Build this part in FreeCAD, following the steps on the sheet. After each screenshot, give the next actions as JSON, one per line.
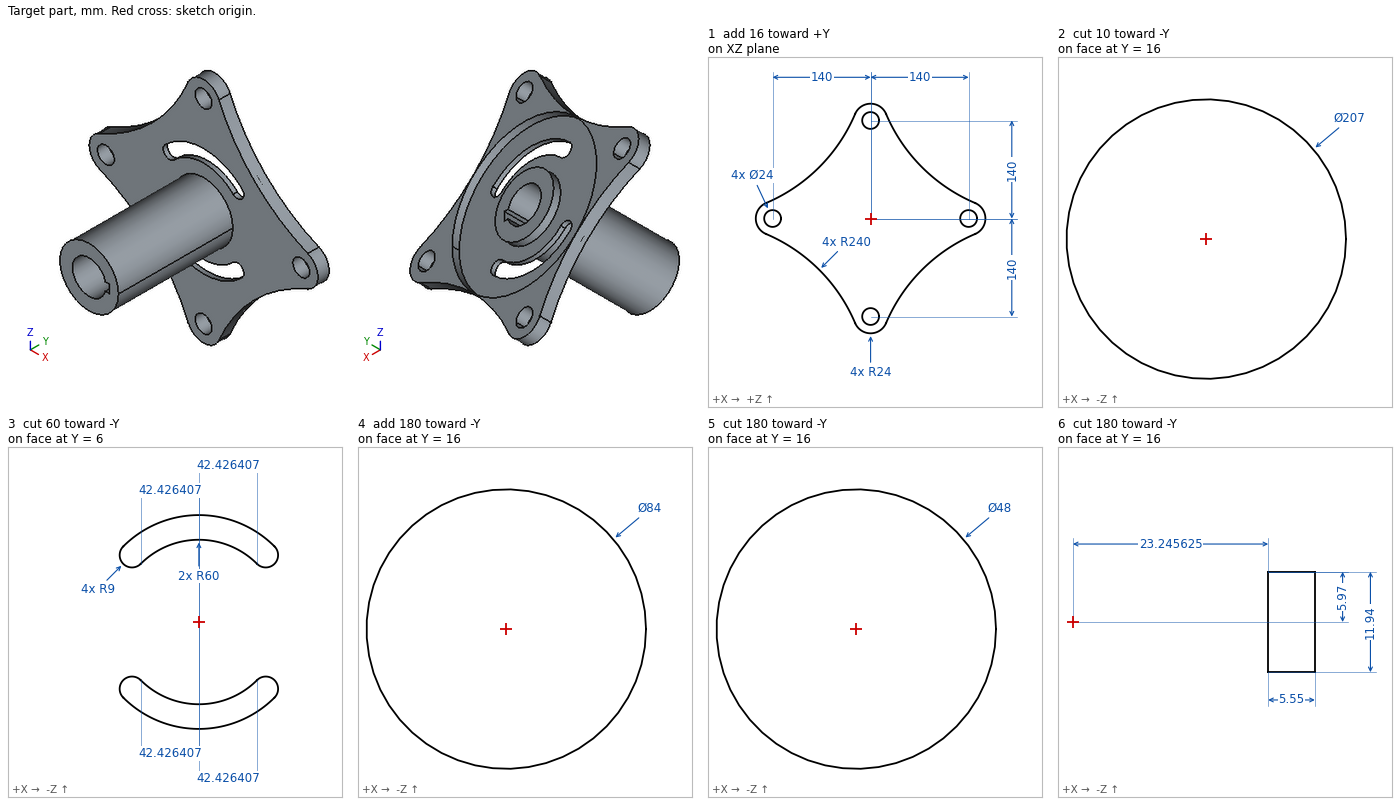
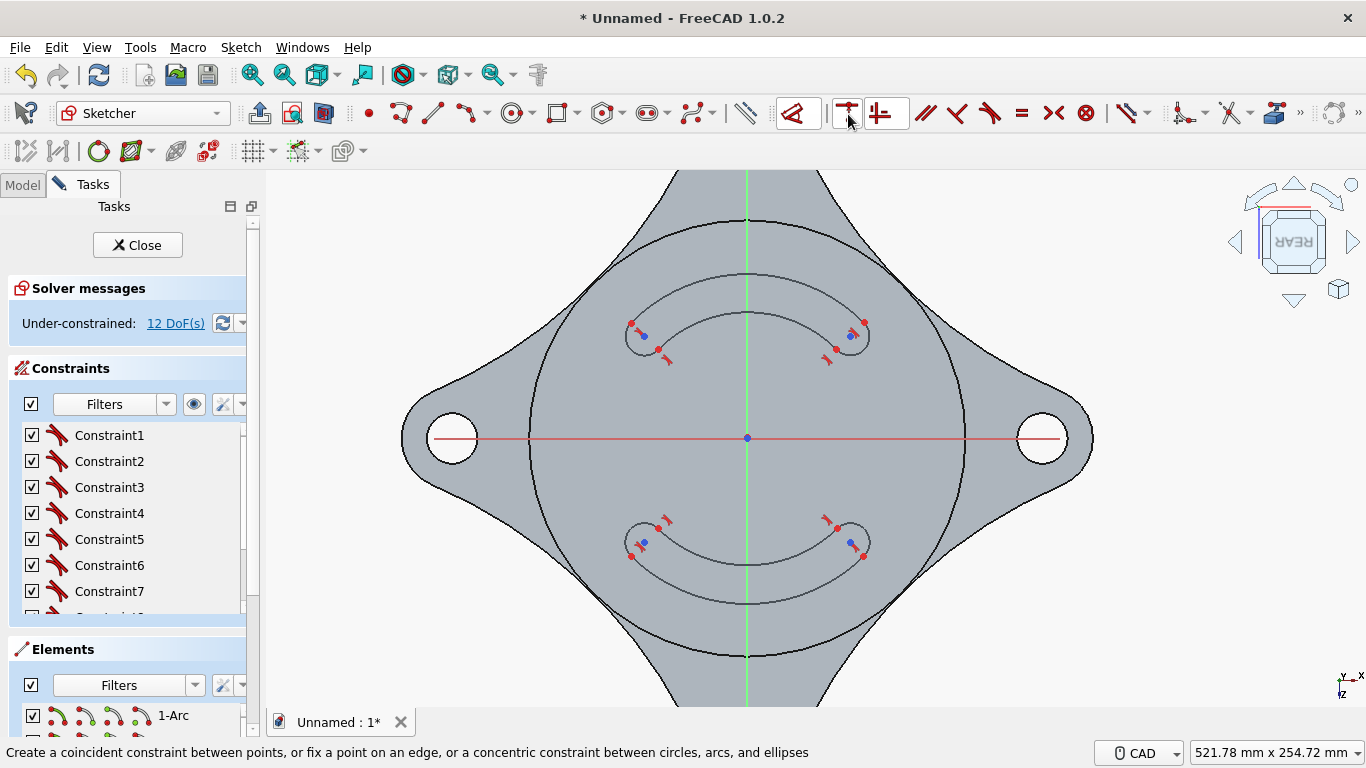
{"action": "left_click", "coordinate": [787, 319]}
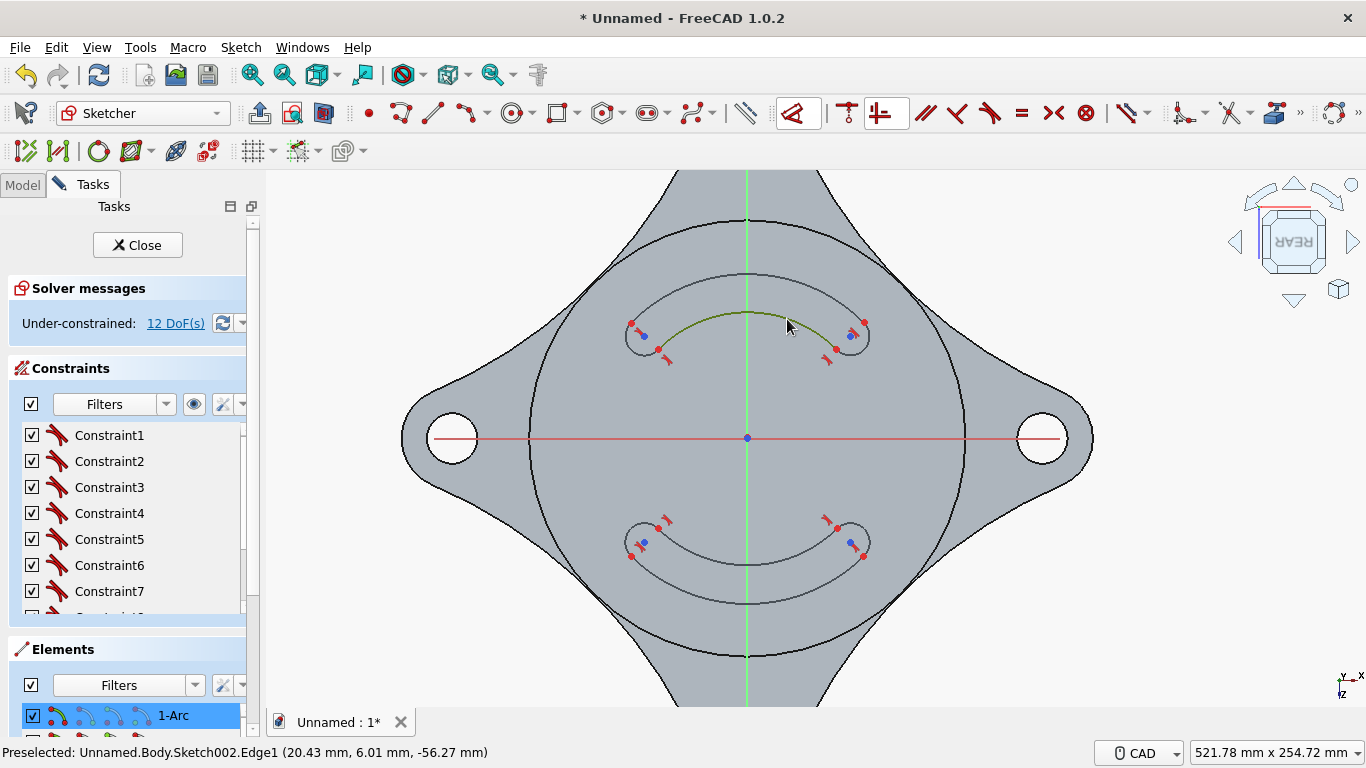
{"action": "left_click", "coordinate": [697, 596]}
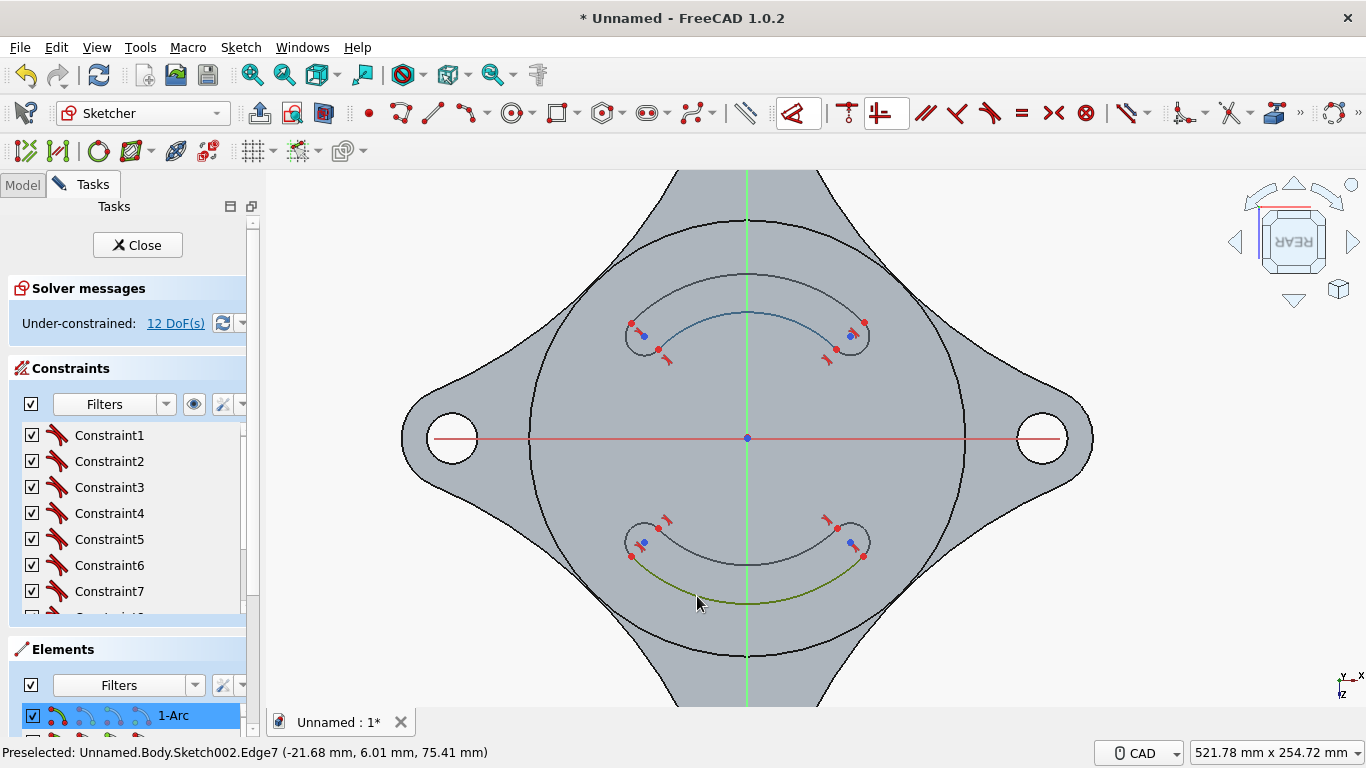
{"action": "left_click", "coordinate": [848, 114]}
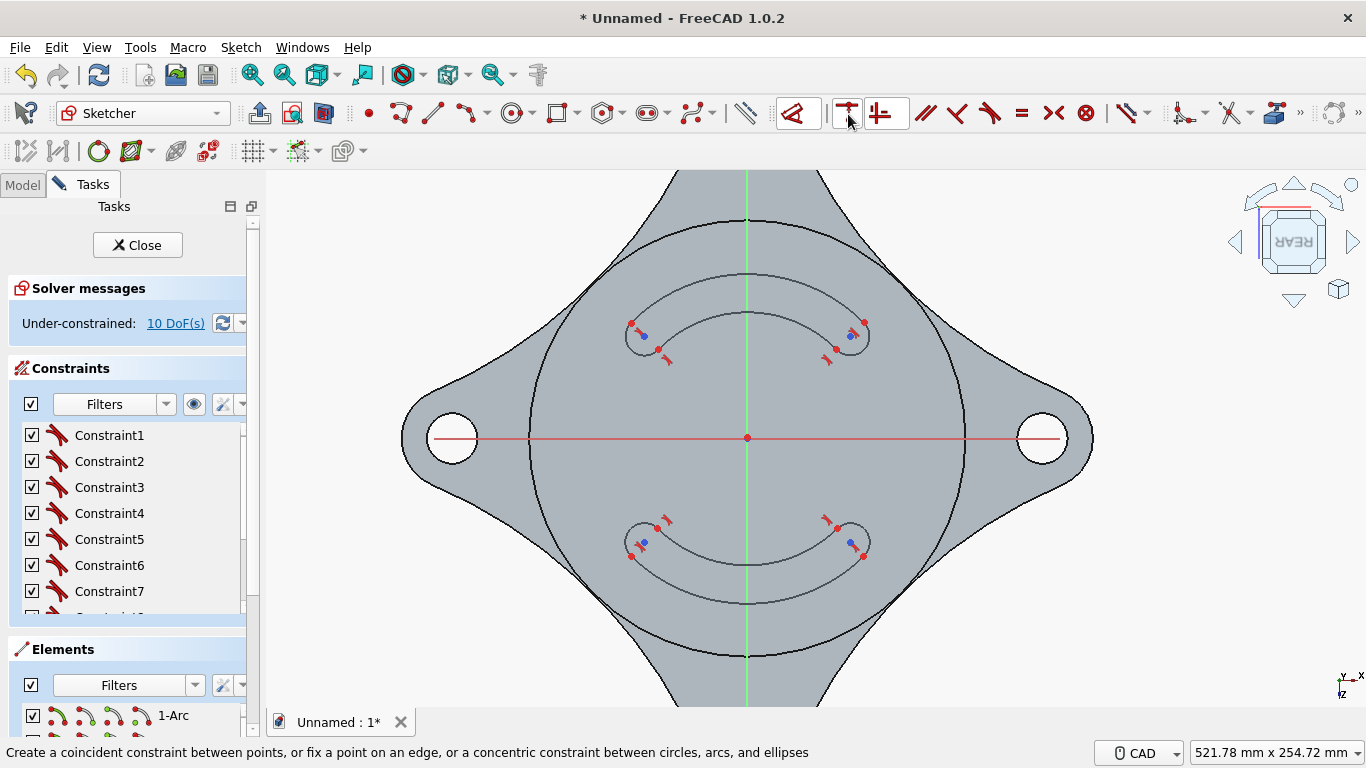
{"action": "scroll", "coordinate": [747, 438], "scroll_direction": "up", "scroll_amount": 4}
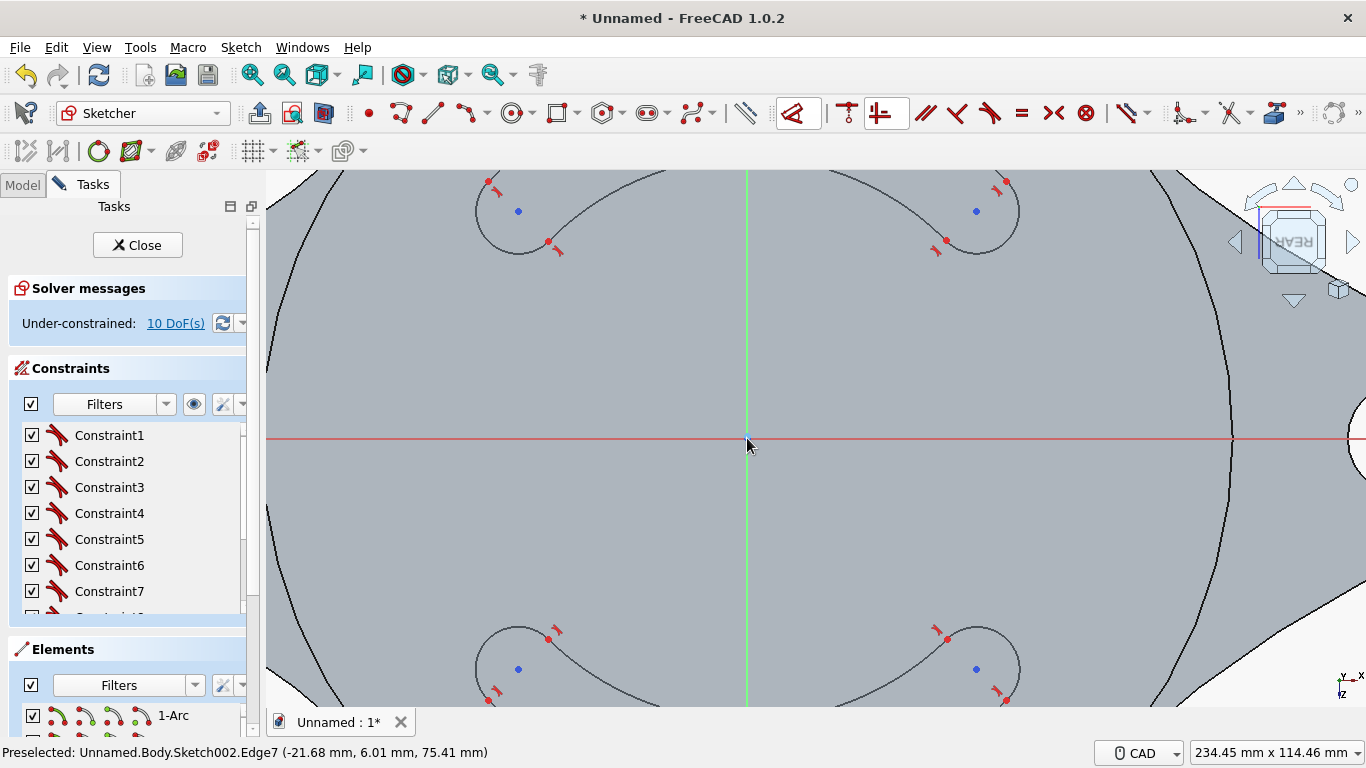
{"action": "left_click_drag", "start_coordinate": [737, 426], "coordinate": [758, 448]}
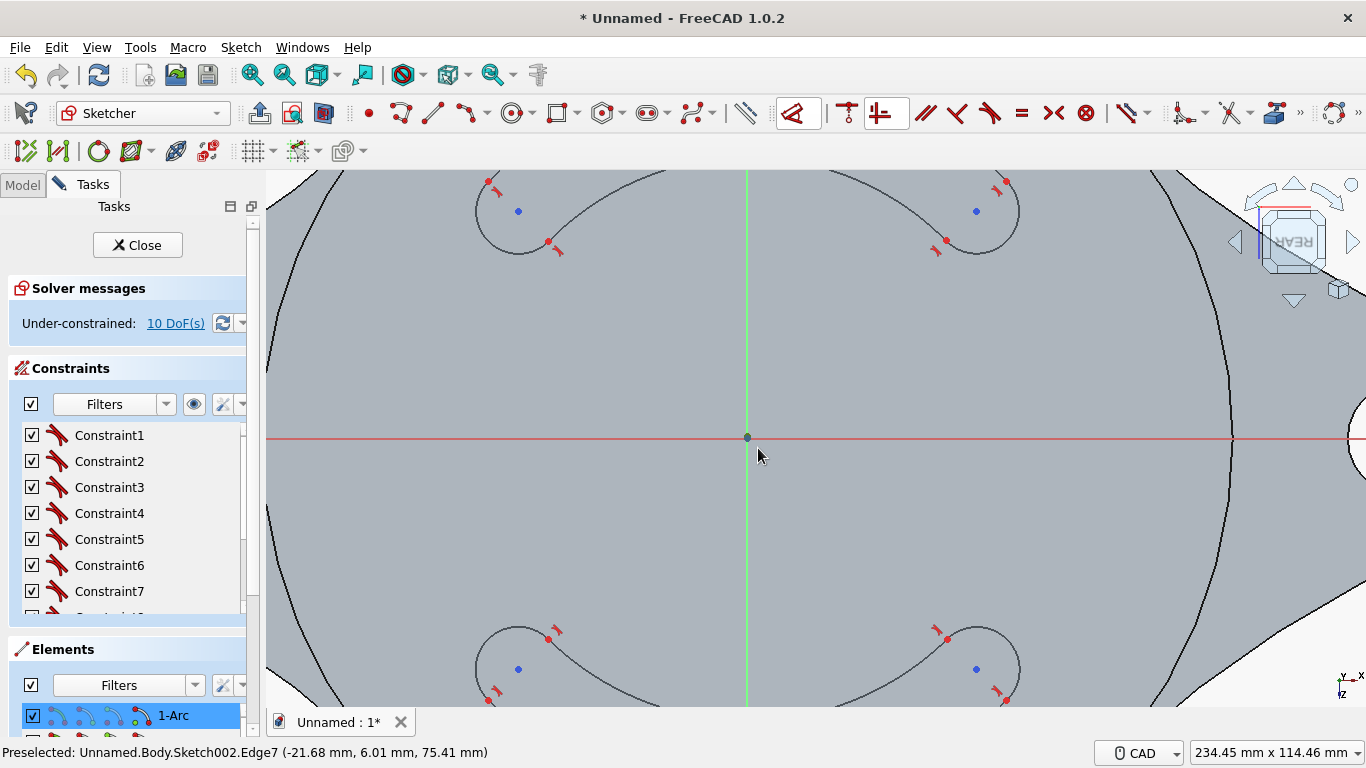
{"action": "left_click", "coordinate": [848, 114]}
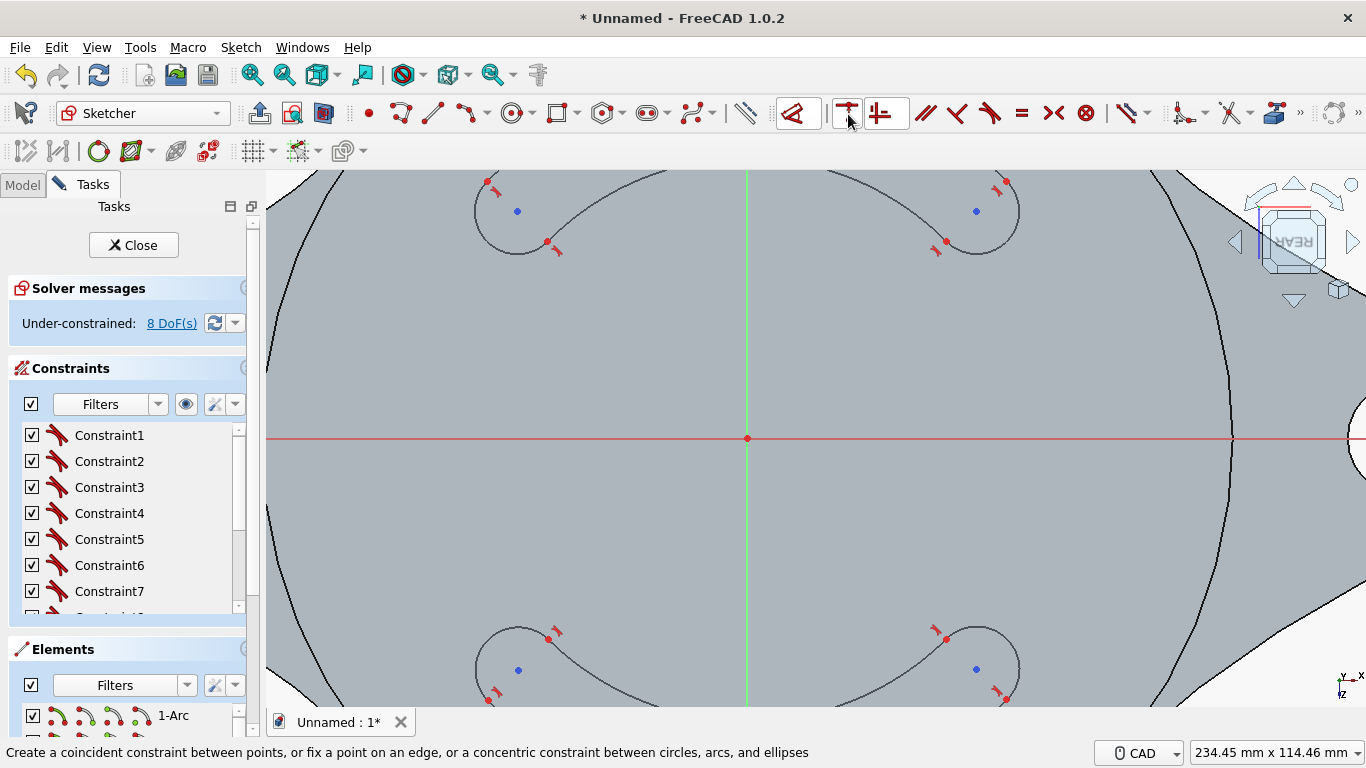
{"action": "scroll", "coordinate": [748, 439], "scroll_direction": "down", "scroll_amount": 4}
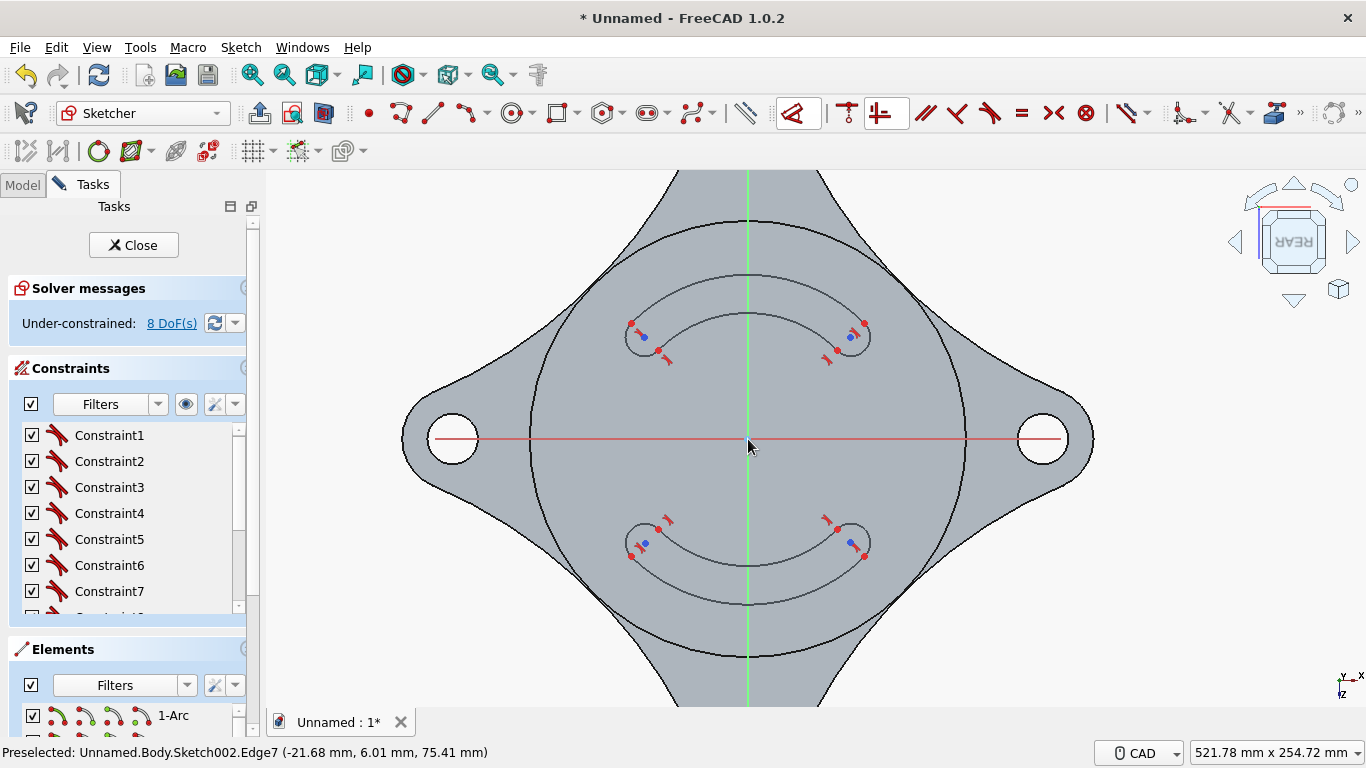
{"action": "left_click", "coordinate": [787, 319]}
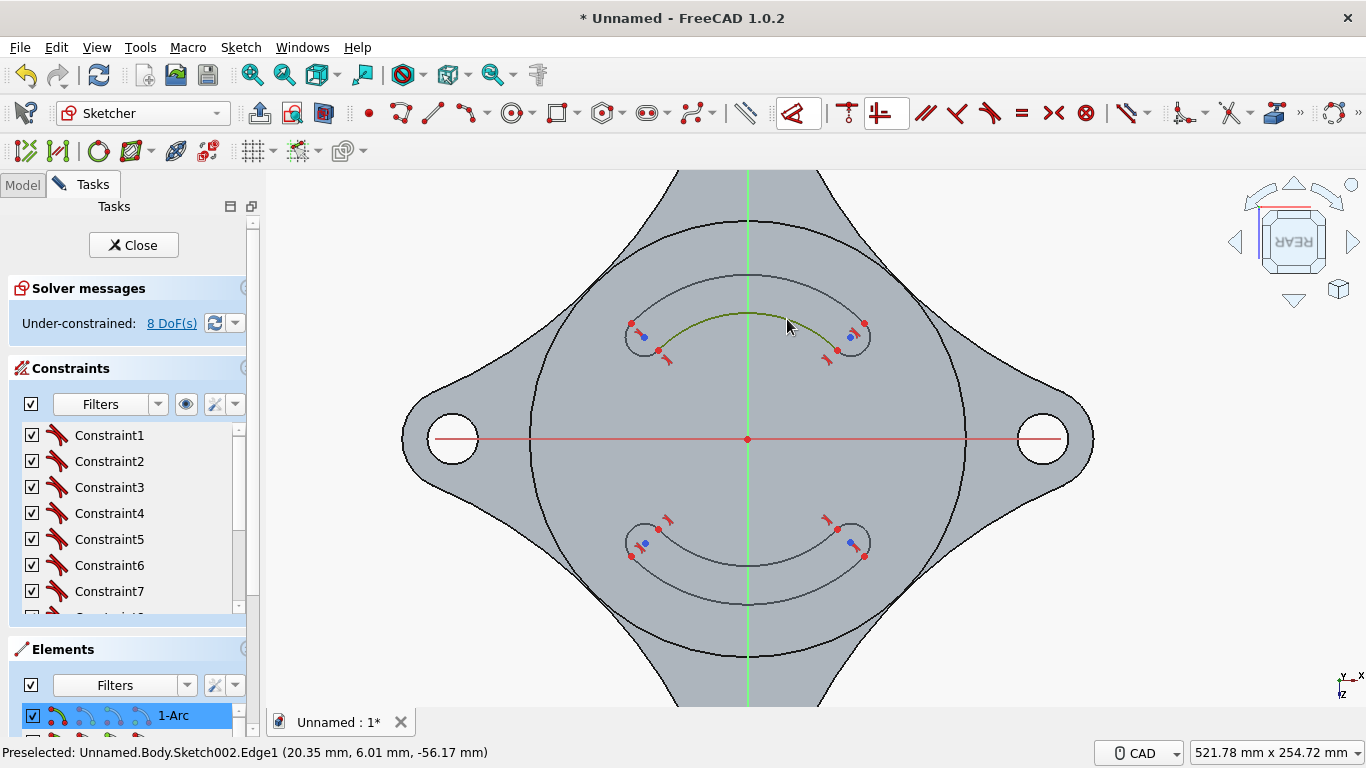
{"action": "left_click", "coordinate": [709, 560]}